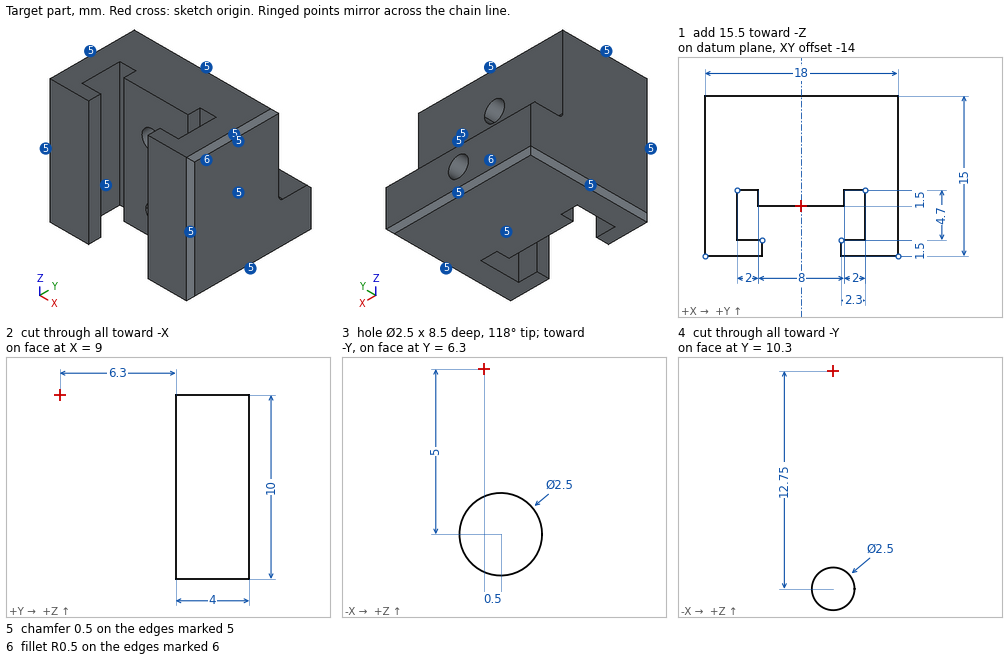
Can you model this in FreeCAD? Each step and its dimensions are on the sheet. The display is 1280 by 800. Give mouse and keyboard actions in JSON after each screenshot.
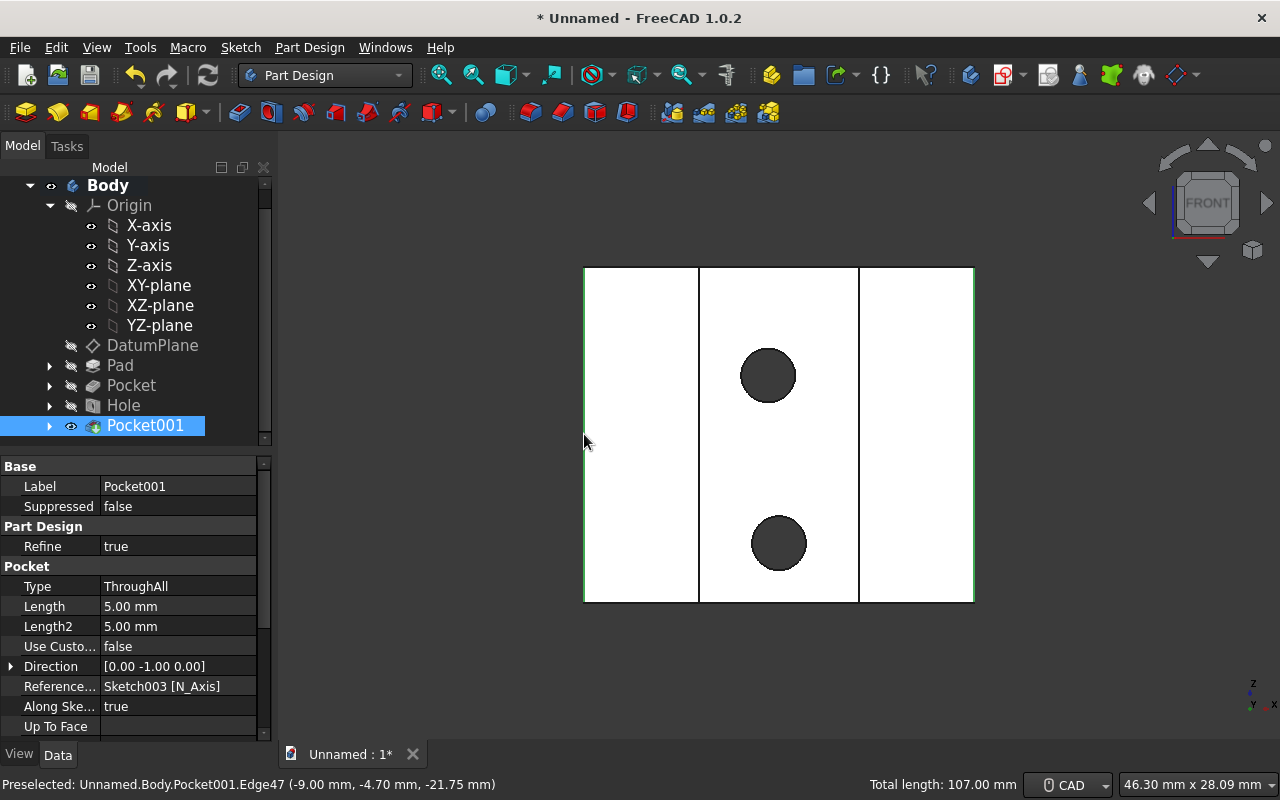
{"action": "key", "text": "3"}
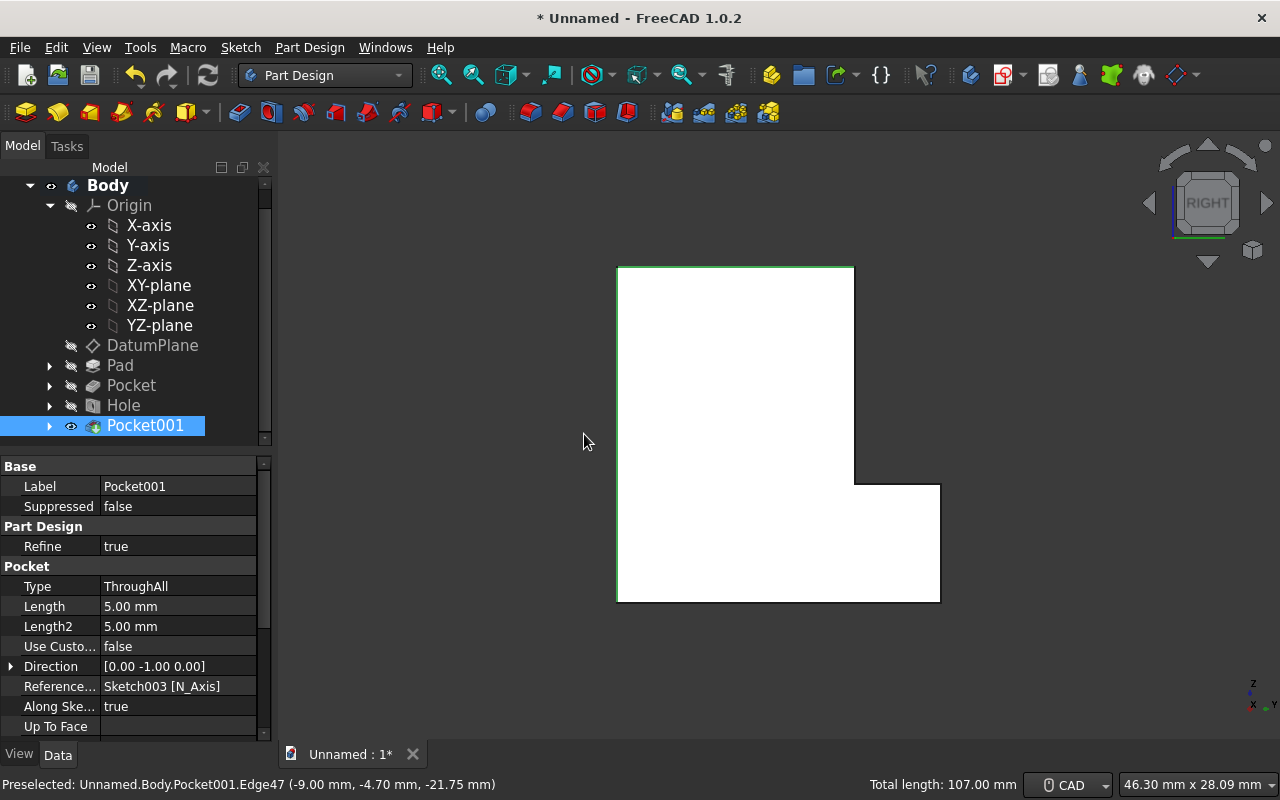
{"action": "left_click", "coordinate": [779, 602], "text": "ctrl"}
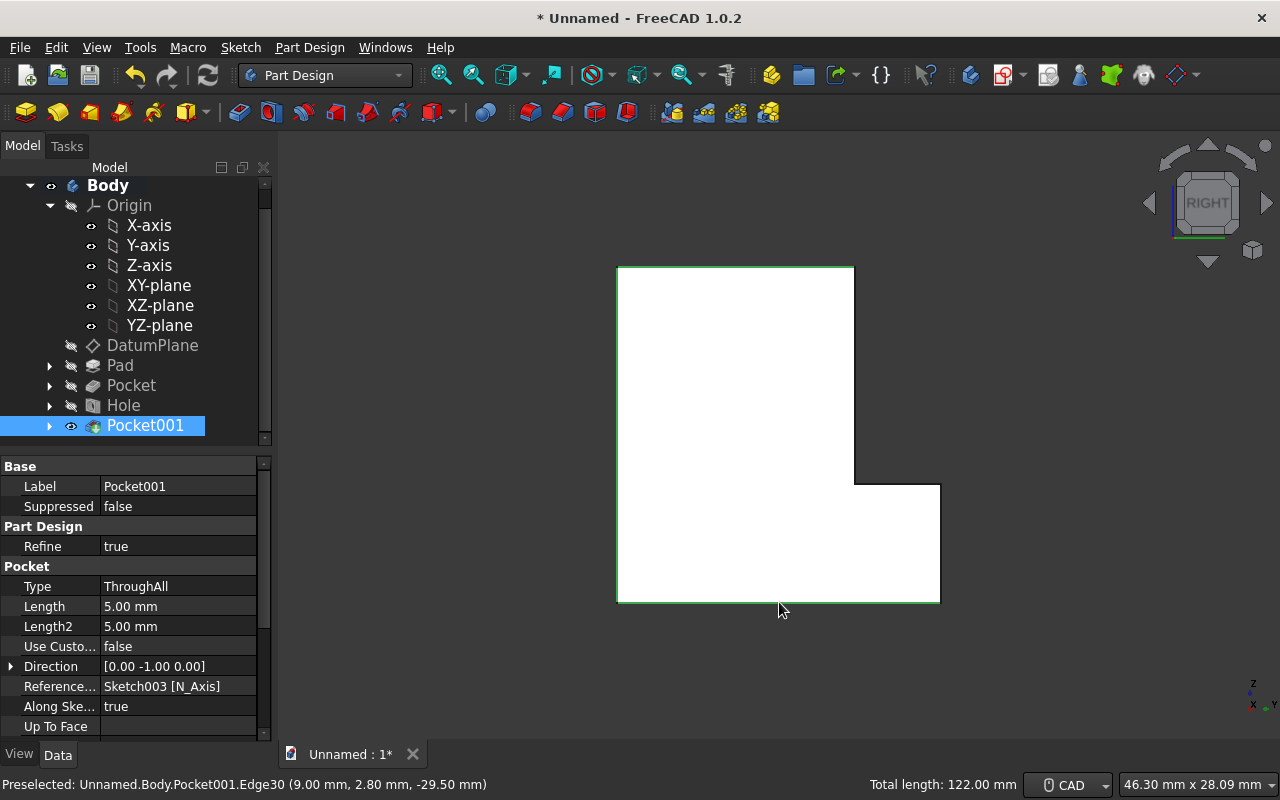
{"action": "key", "text": "5"}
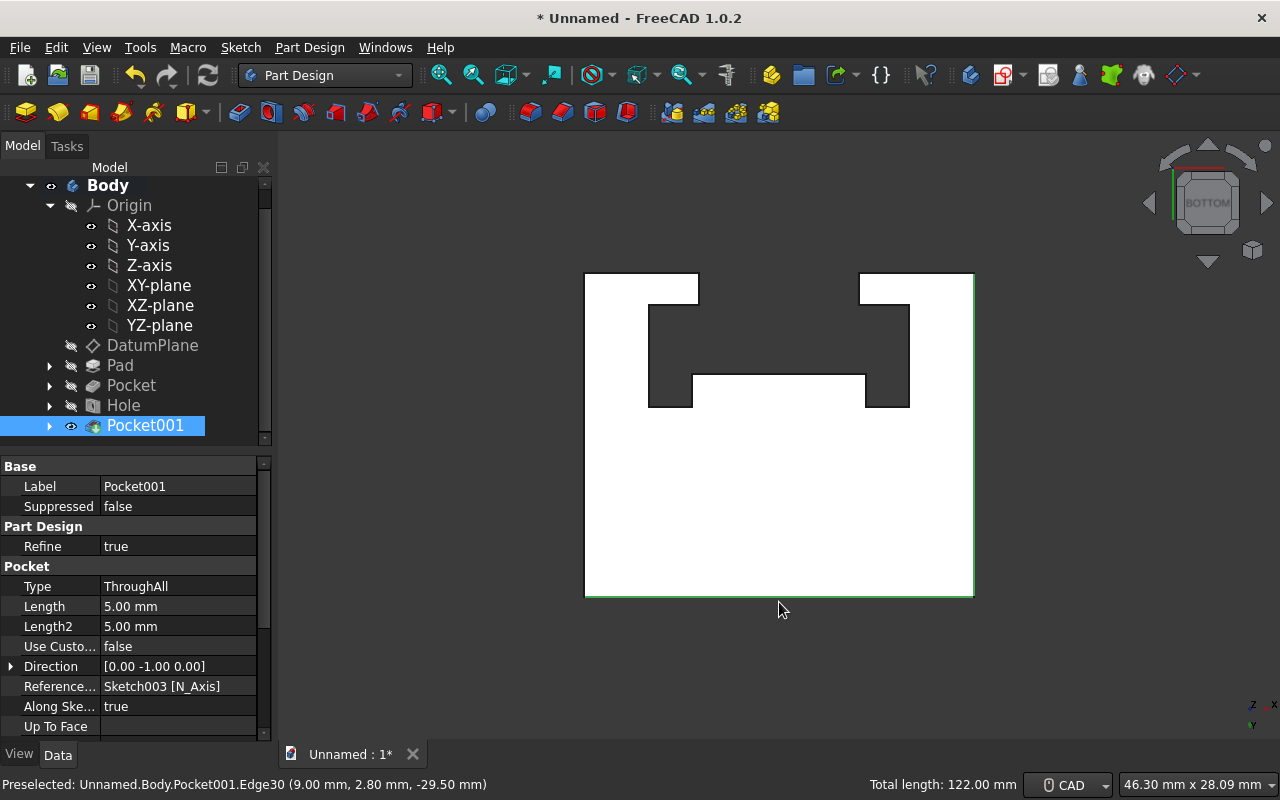
{"action": "left_click", "coordinate": [584, 434], "text": "ctrl"}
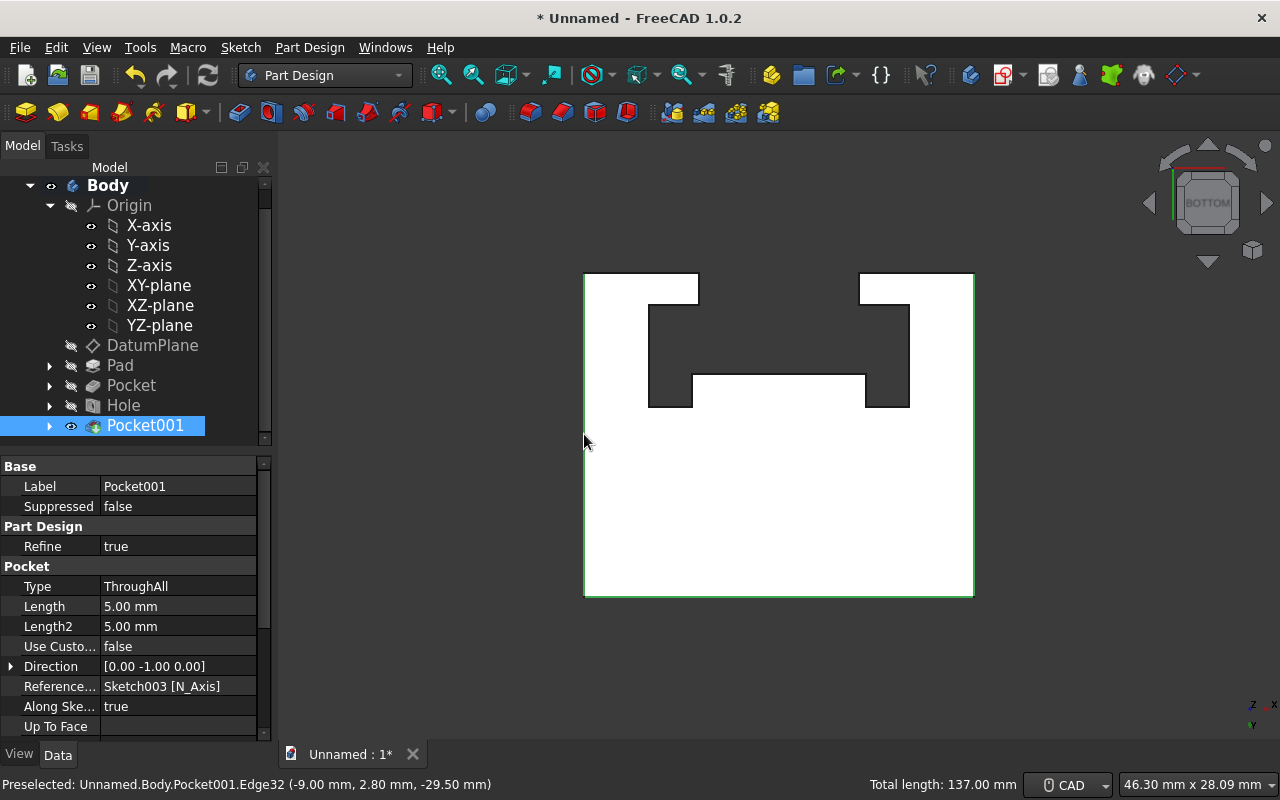
{"action": "left_click", "coordinate": [564, 112]}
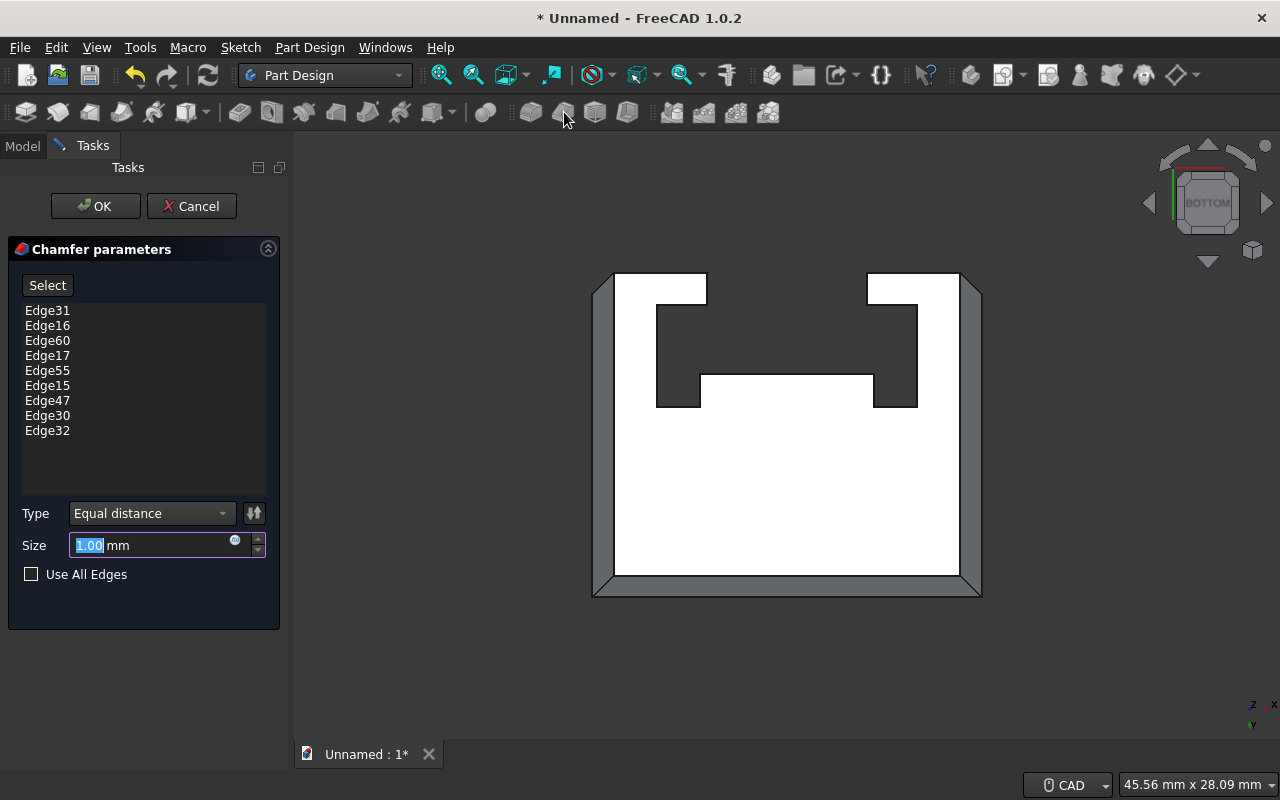
{"action": "type", "text": "0.5"}
{"action": "key", "text": "Tab"}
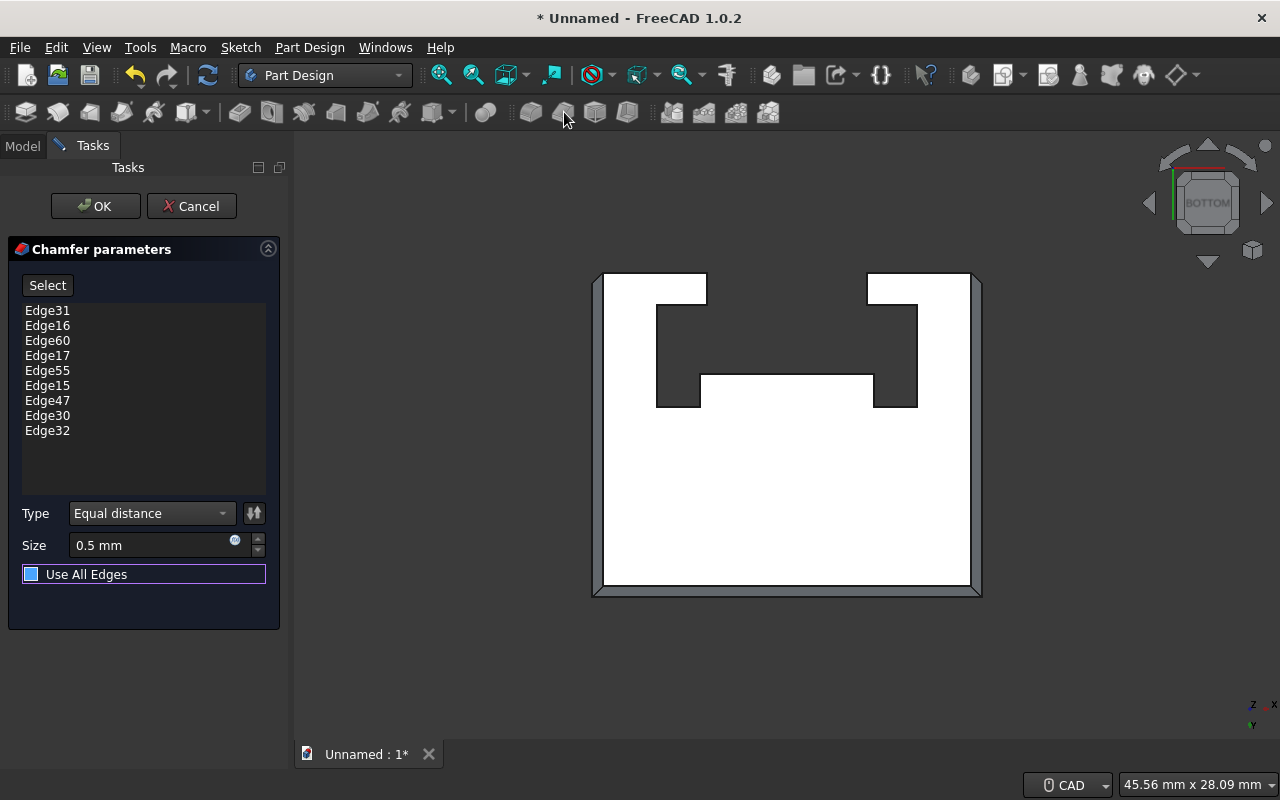
{"action": "left_click", "coordinate": [96, 206]}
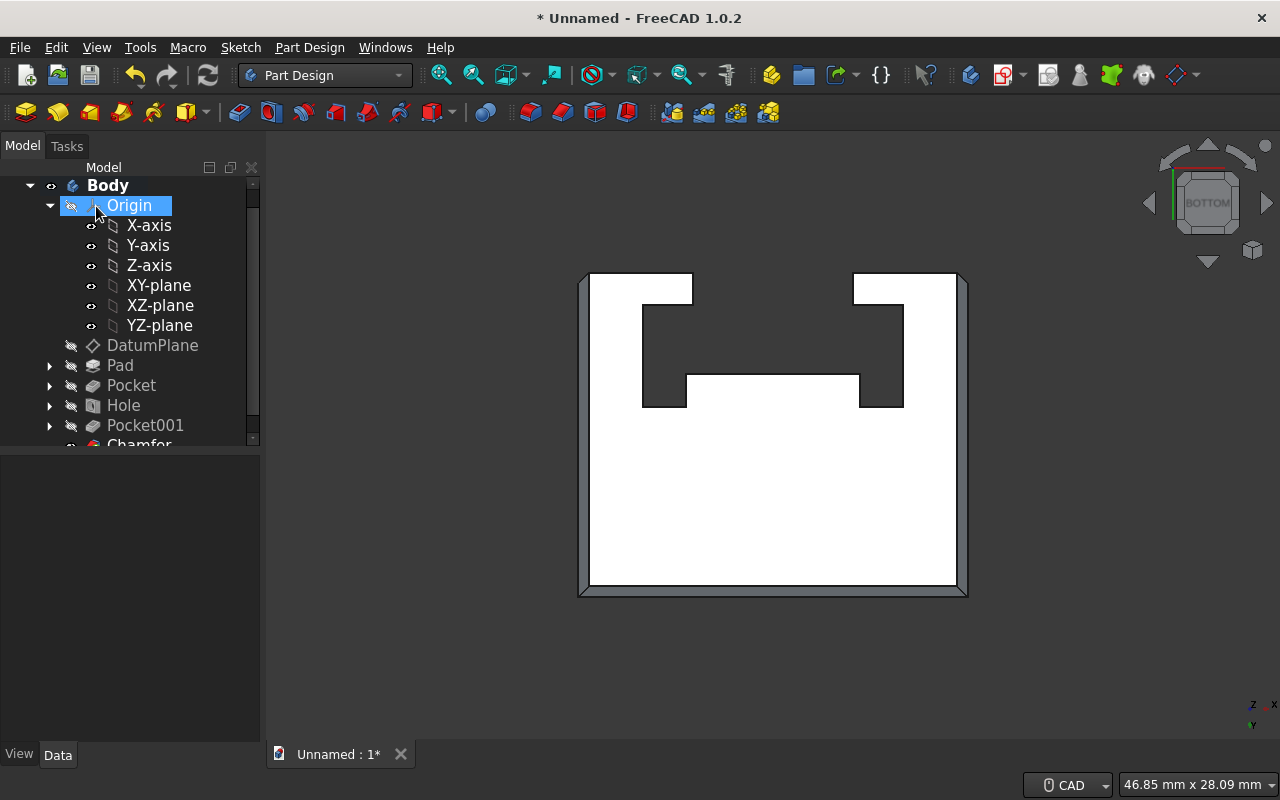
{"action": "key", "text": "0"}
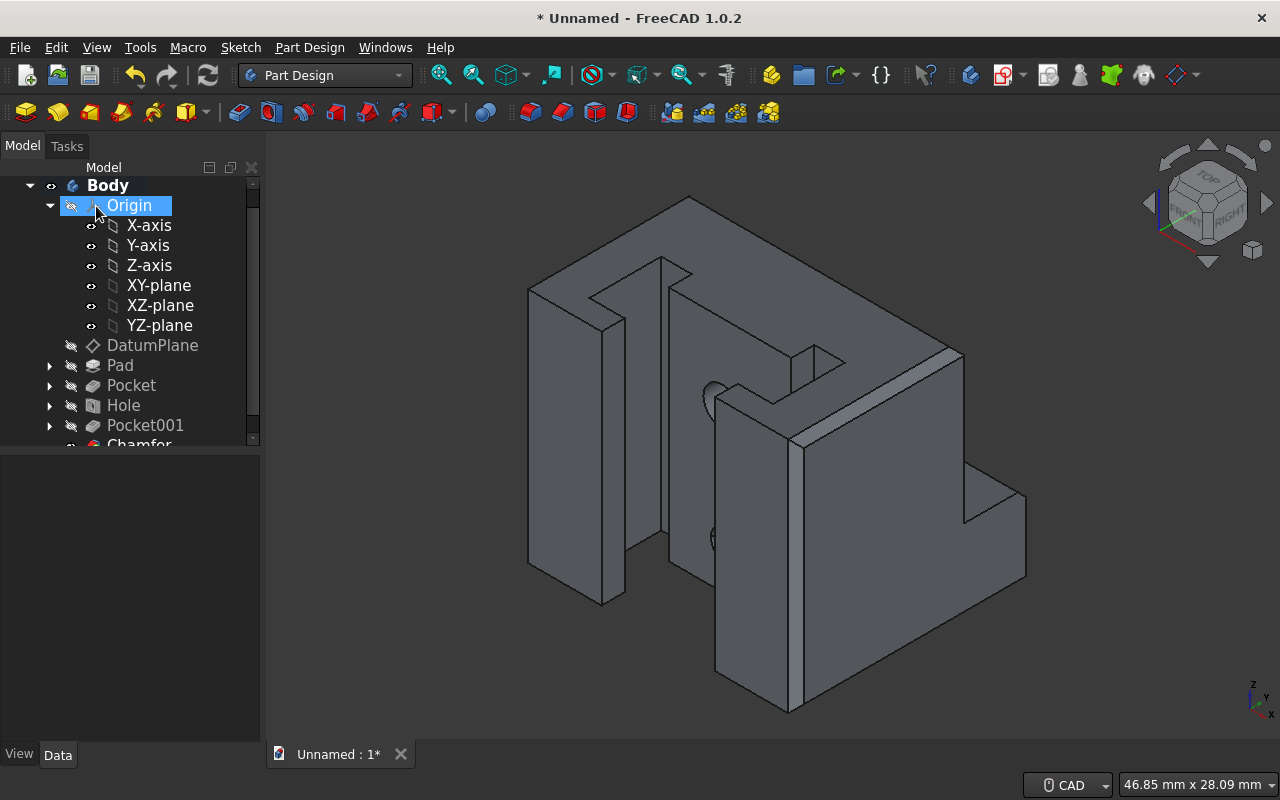
{"action": "key", "text": "2"}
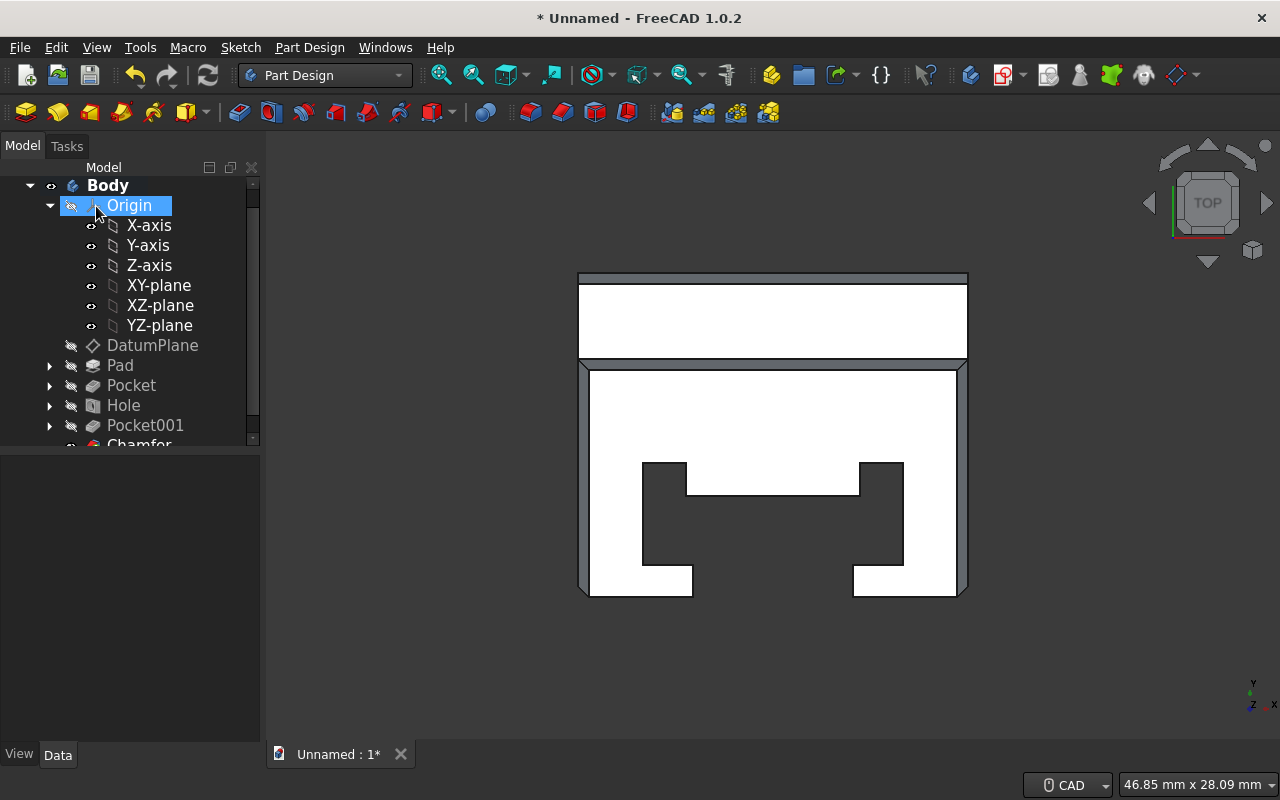
{"action": "key", "text": "1"}